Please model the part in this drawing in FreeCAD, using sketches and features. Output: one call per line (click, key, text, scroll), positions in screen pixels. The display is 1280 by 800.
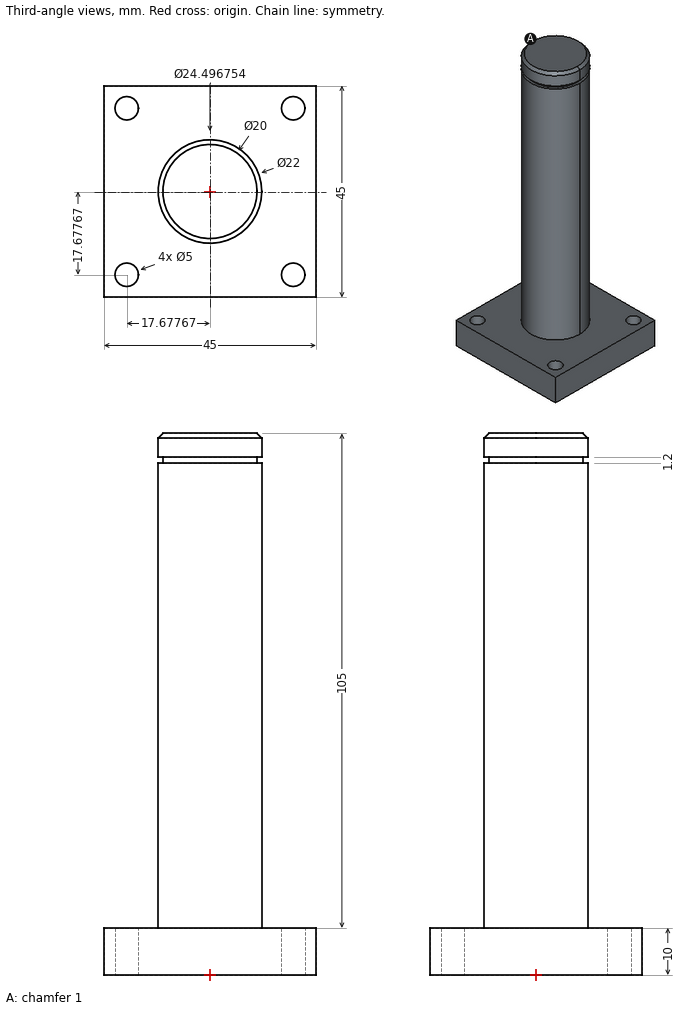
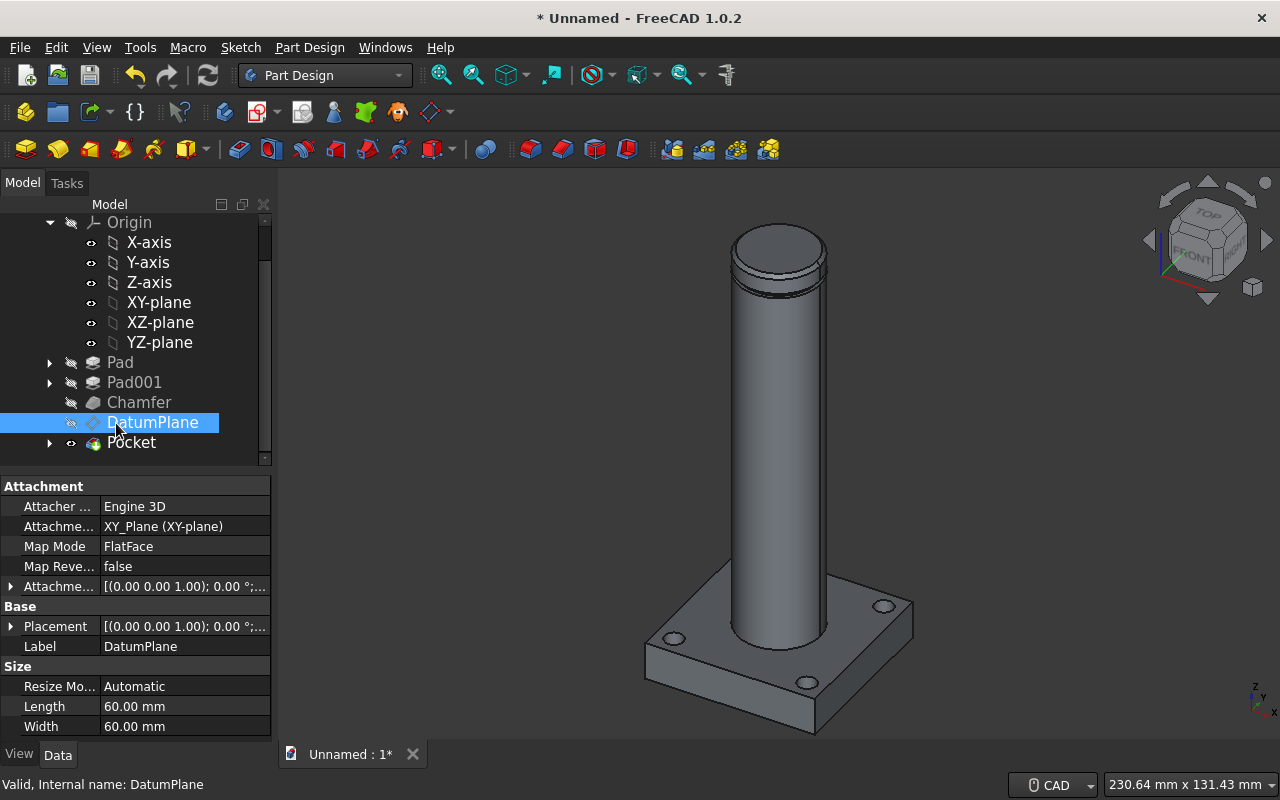
key(0)